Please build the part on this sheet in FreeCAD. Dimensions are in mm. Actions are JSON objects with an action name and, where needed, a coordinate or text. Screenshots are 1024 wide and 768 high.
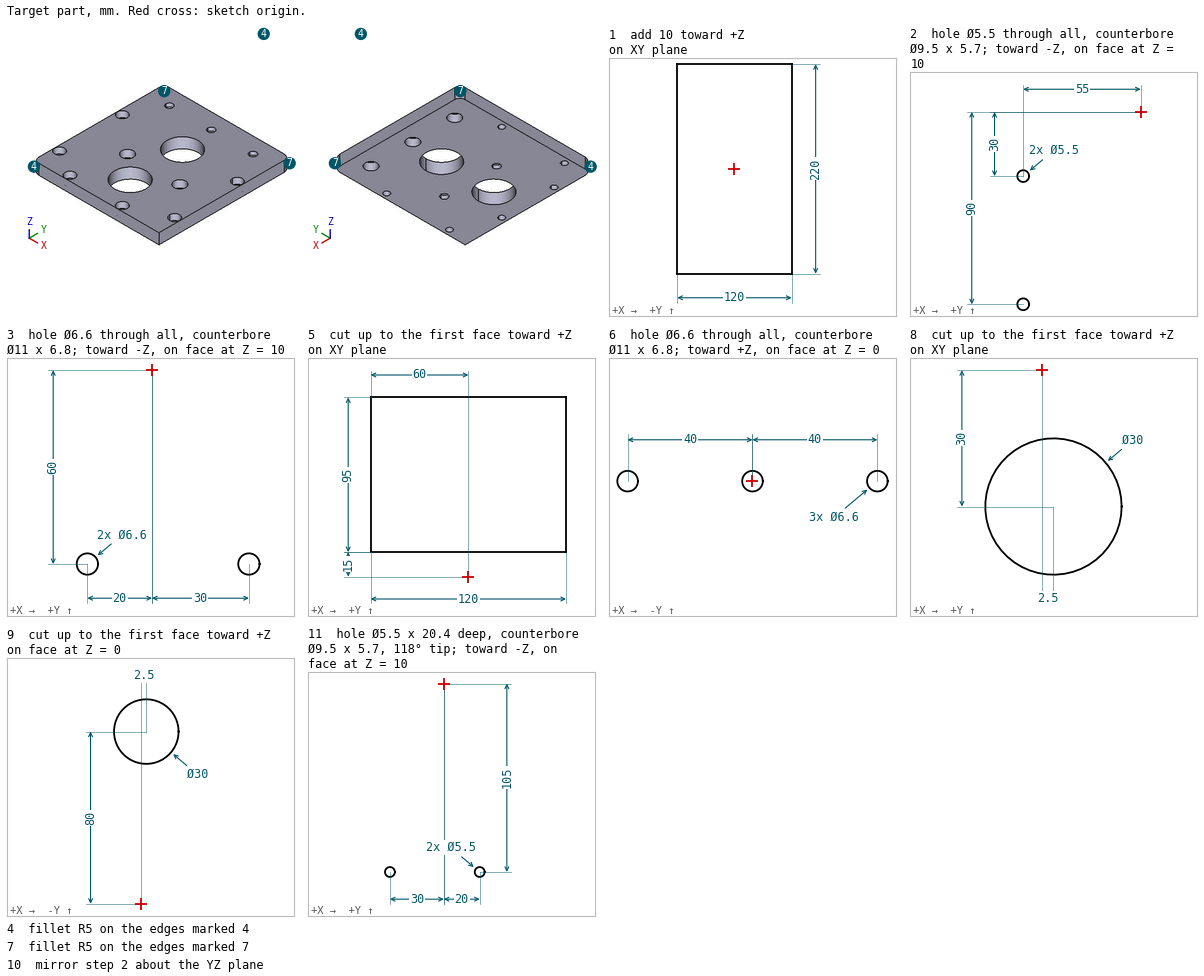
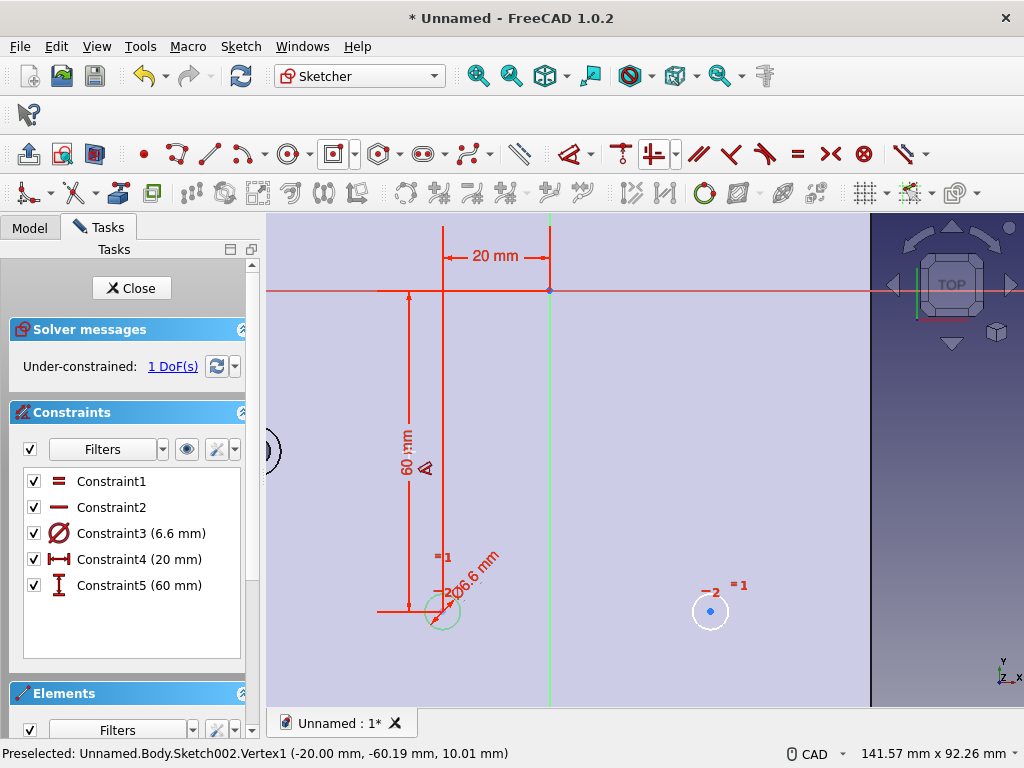
{"action": "left_click", "coordinate": [711, 612]}
{"action": "left_click", "coordinate": [630, 257]}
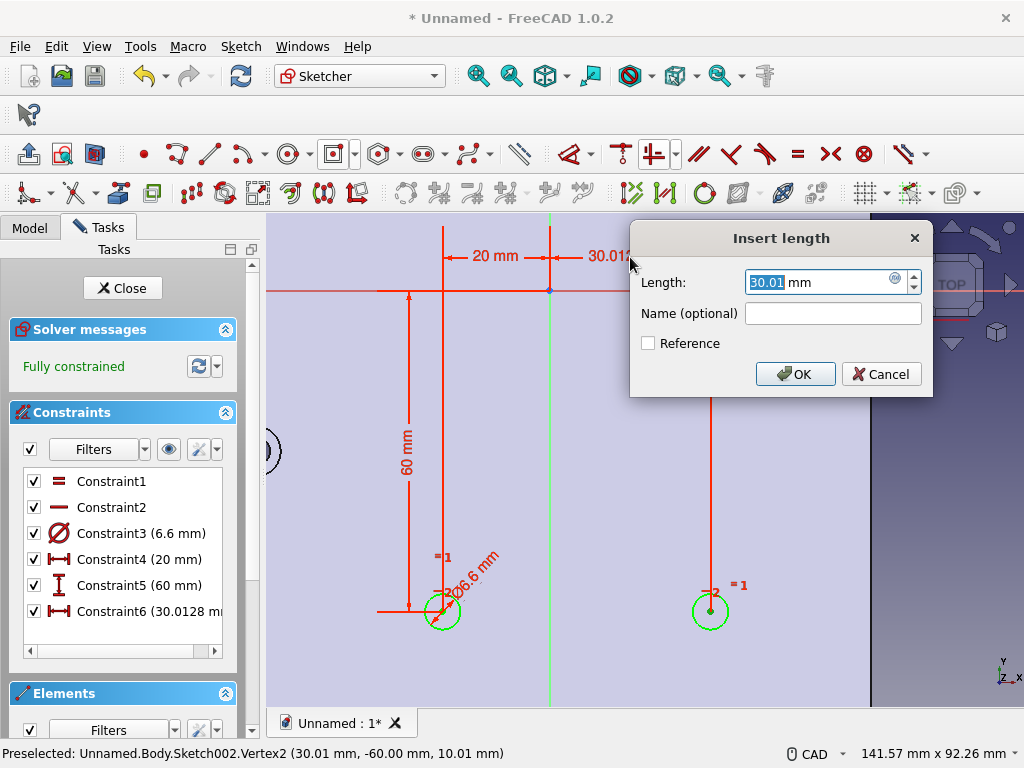
{"action": "type", "text": "30"}
{"action": "key", "text": "Return"}
{"action": "key", "text": "Escape"}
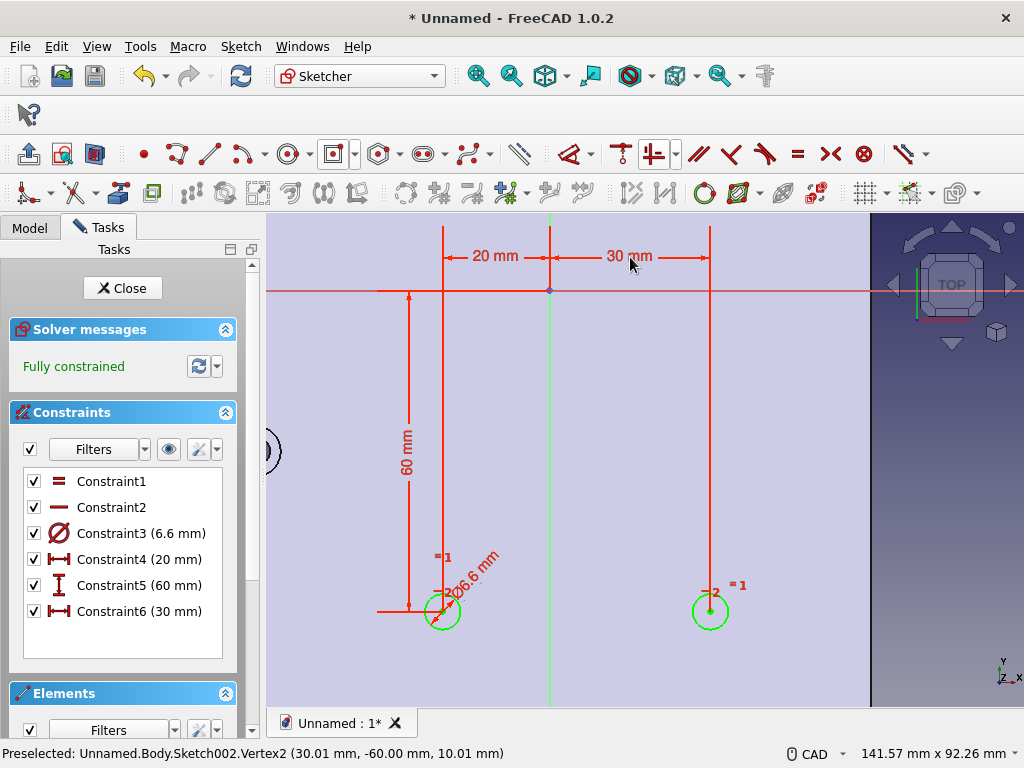
{"action": "left_click", "coordinate": [123, 288]}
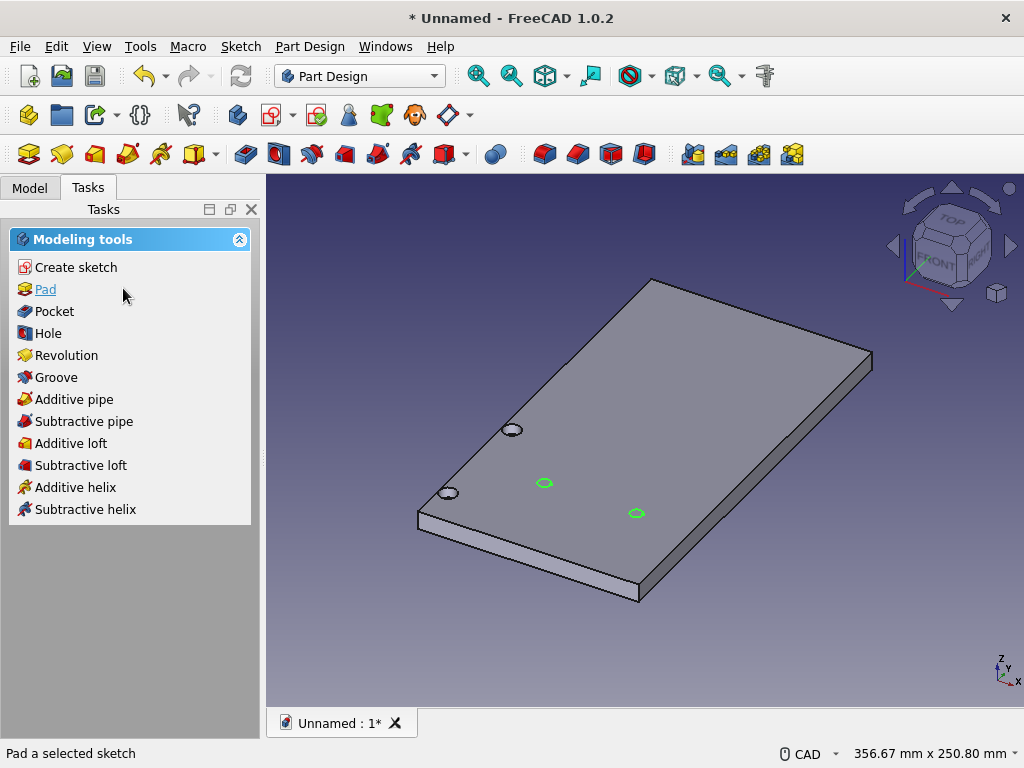
{"action": "left_click", "coordinate": [279, 154]}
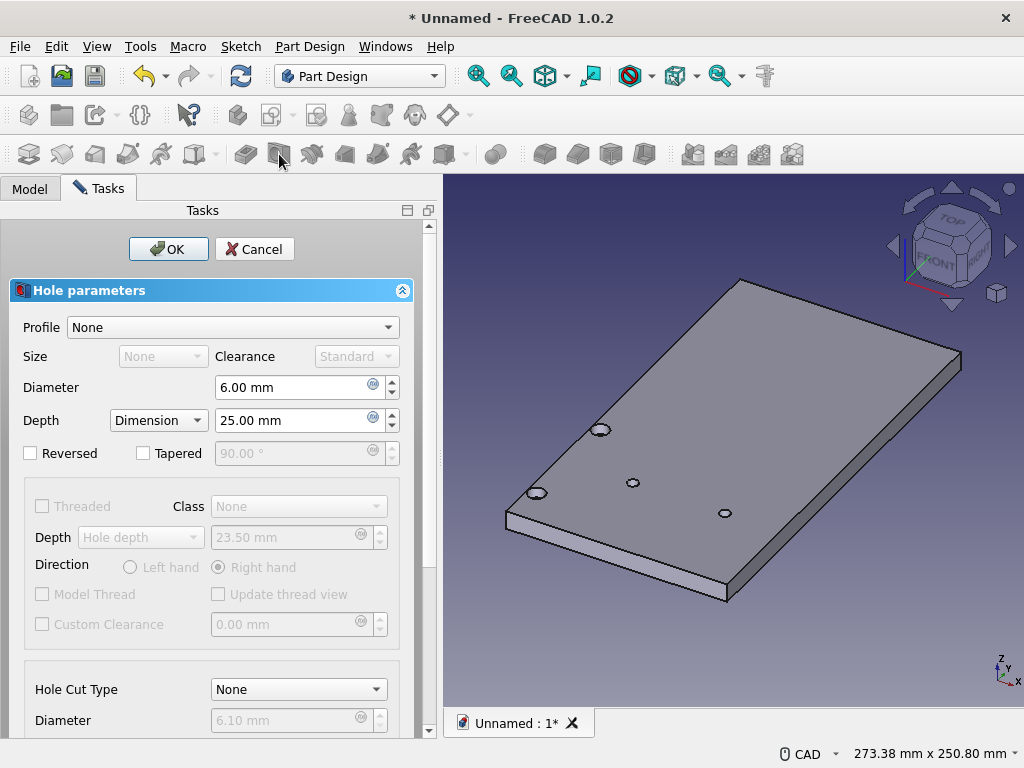
{"action": "triple_click", "coordinate": [300, 388]}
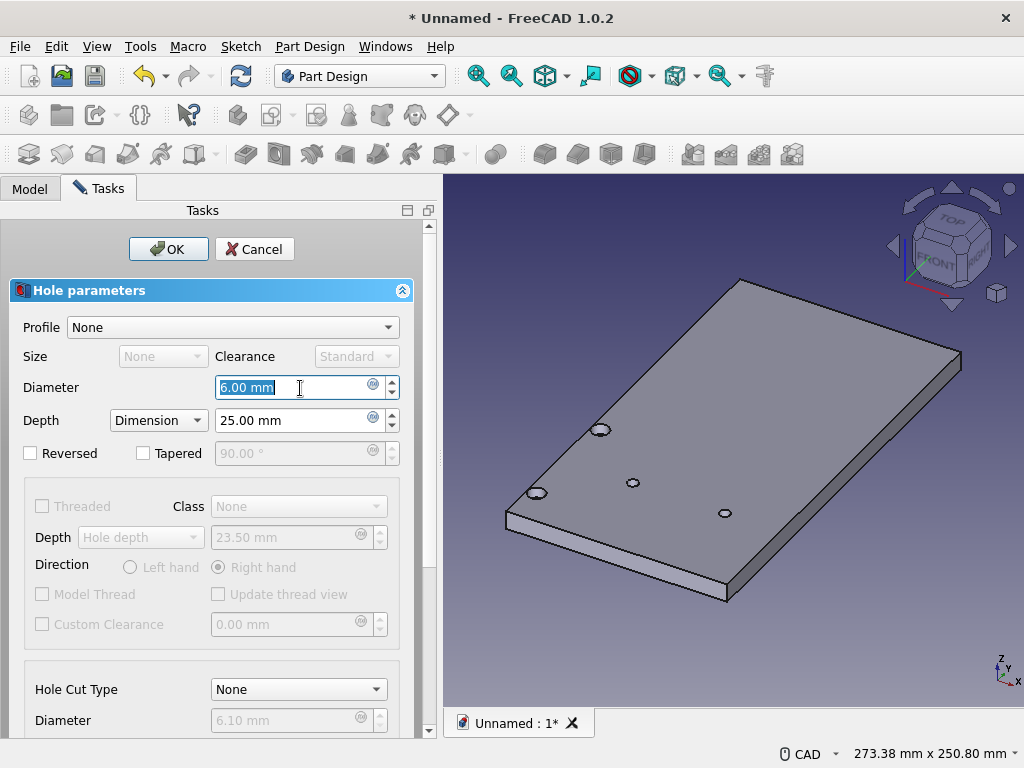
{"action": "type", "text": "6.6"}
{"action": "key", "text": "Tab"}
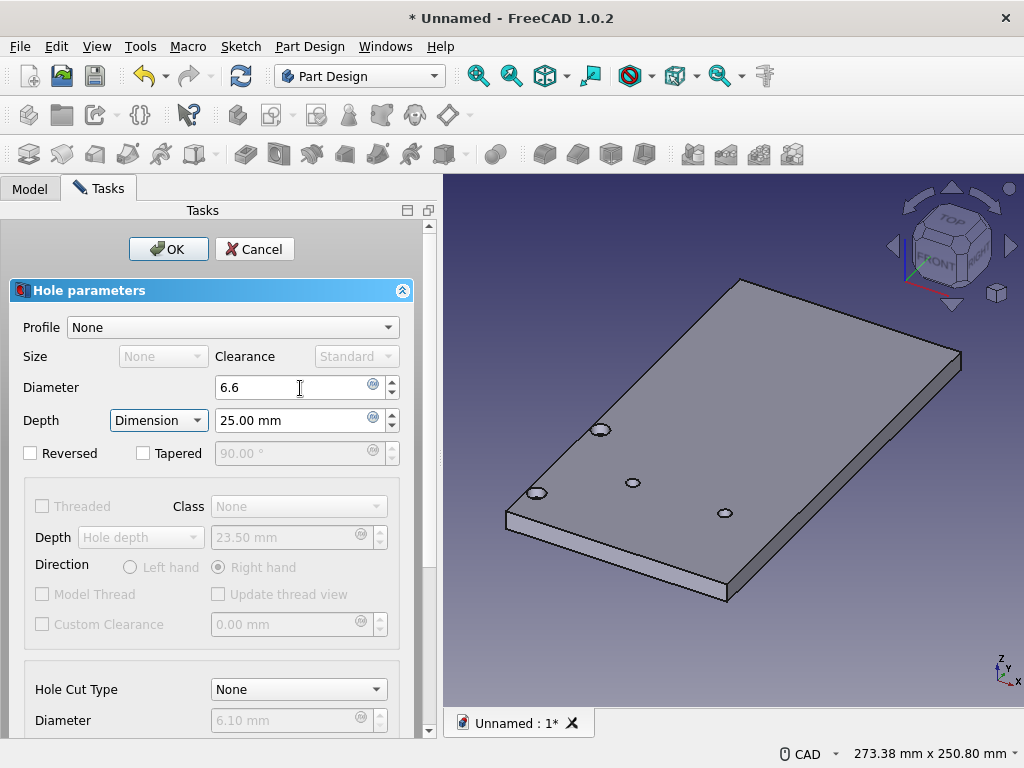
{"action": "left_click", "coordinate": [160, 420]}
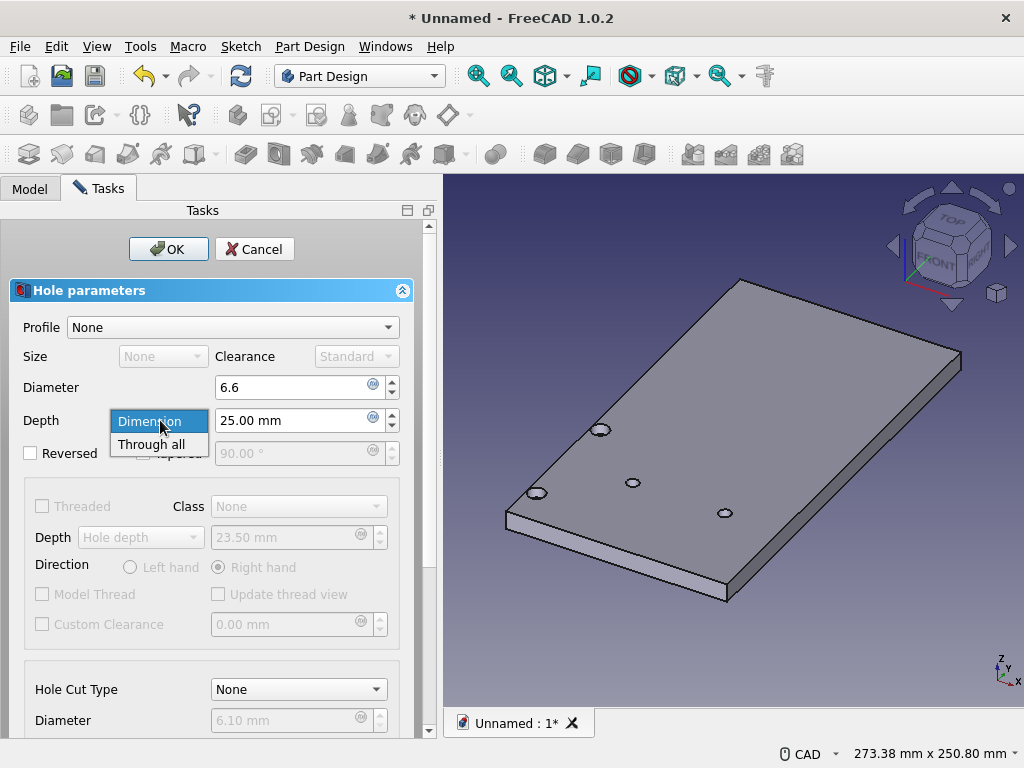
{"action": "left_click", "coordinate": [158, 444]}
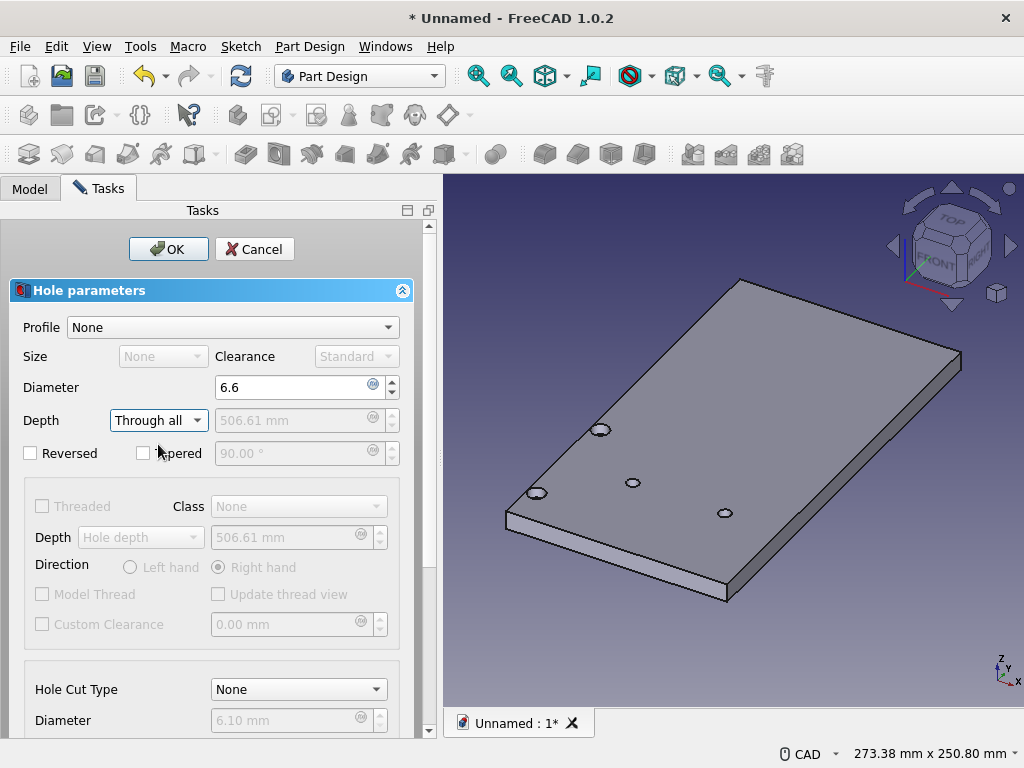
{"action": "left_click", "coordinate": [300, 690]}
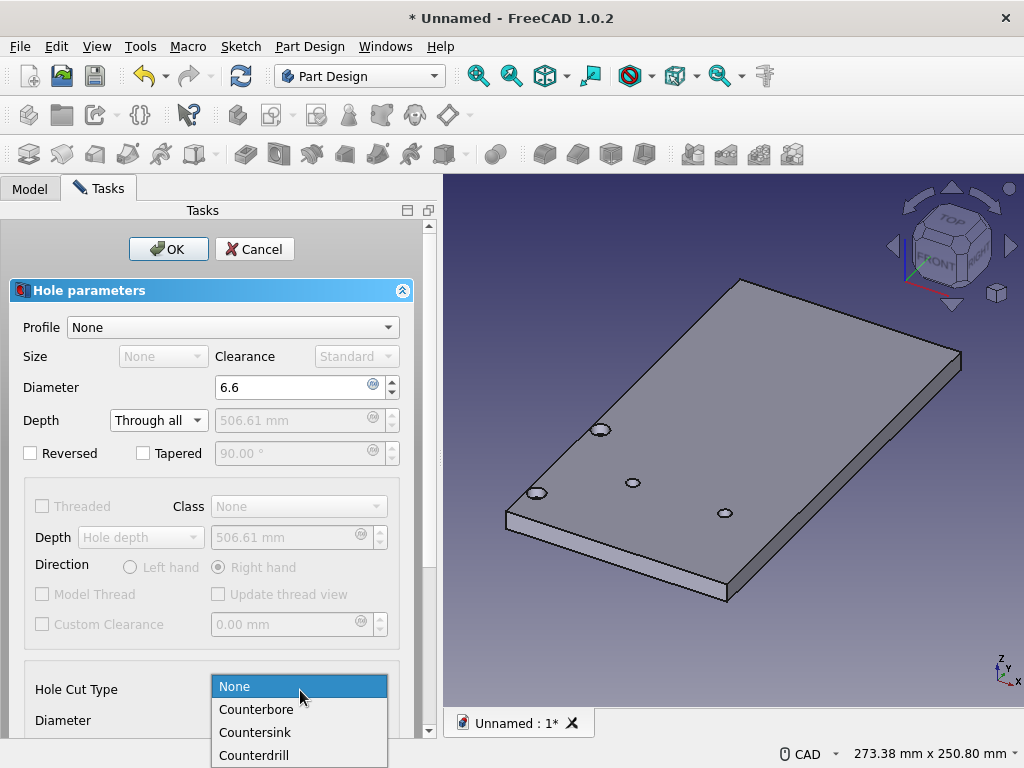
{"action": "left_click", "coordinate": [298, 710]}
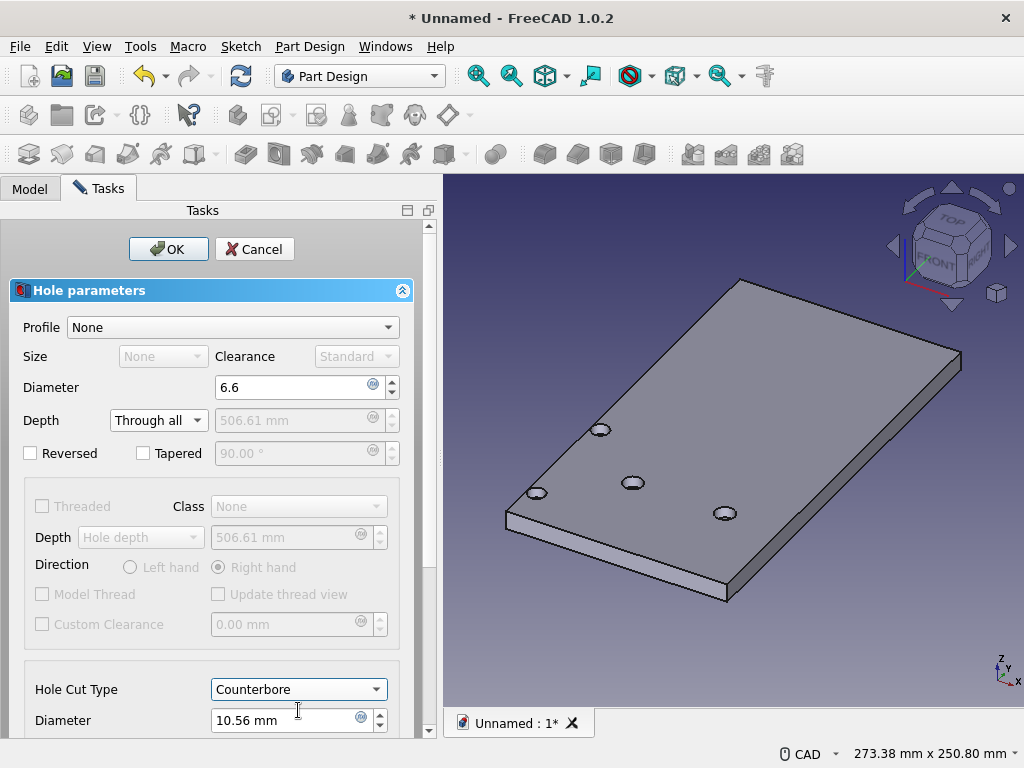
{"action": "triple_click", "coordinate": [292, 720]}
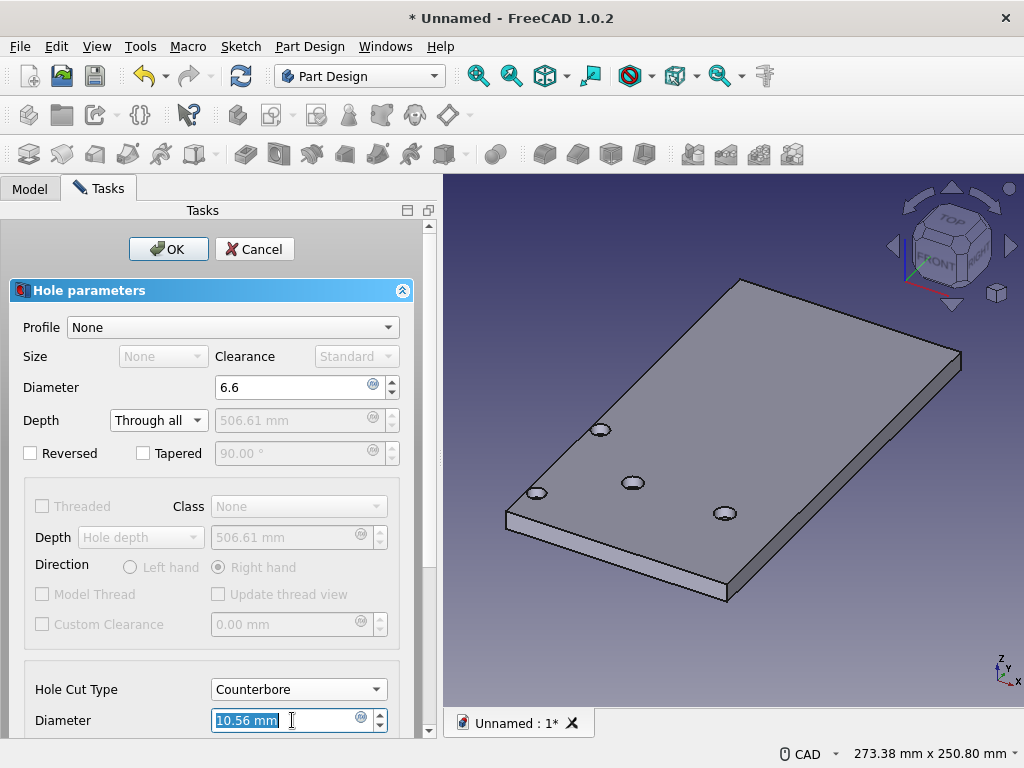
{"action": "type", "text": "11"}
{"action": "key", "text": "Tab"}